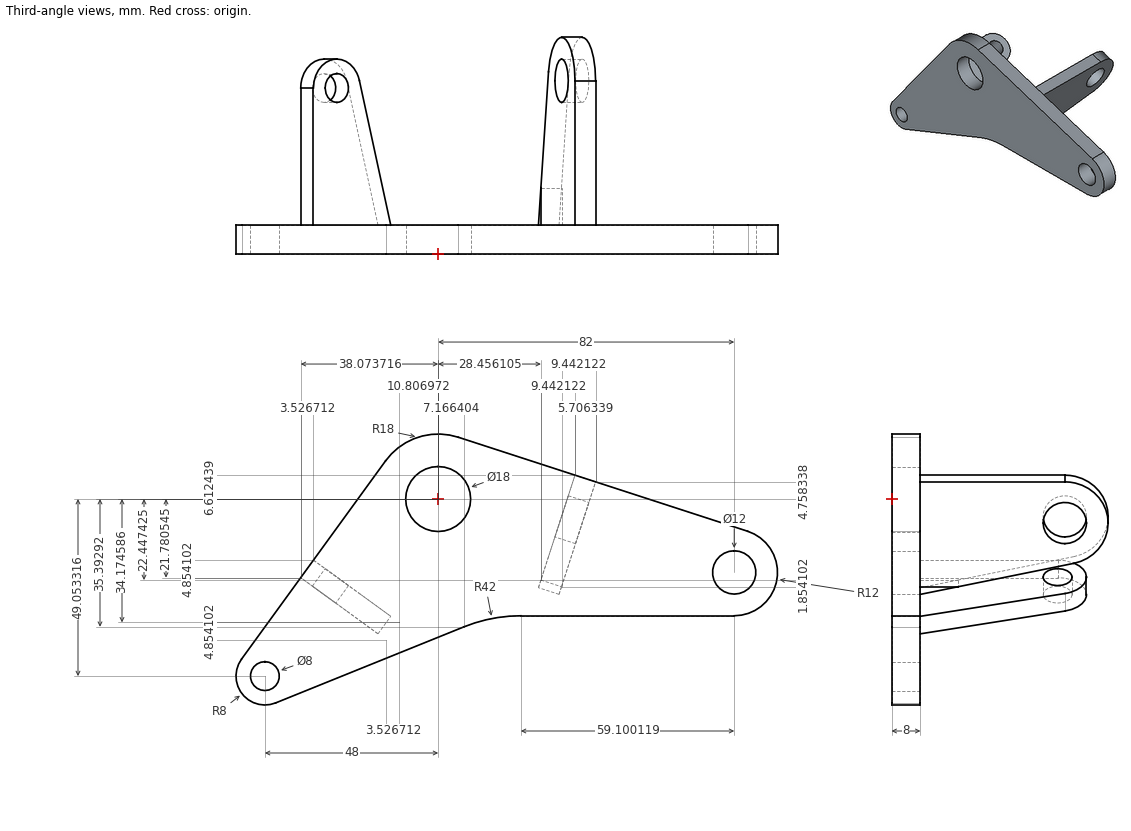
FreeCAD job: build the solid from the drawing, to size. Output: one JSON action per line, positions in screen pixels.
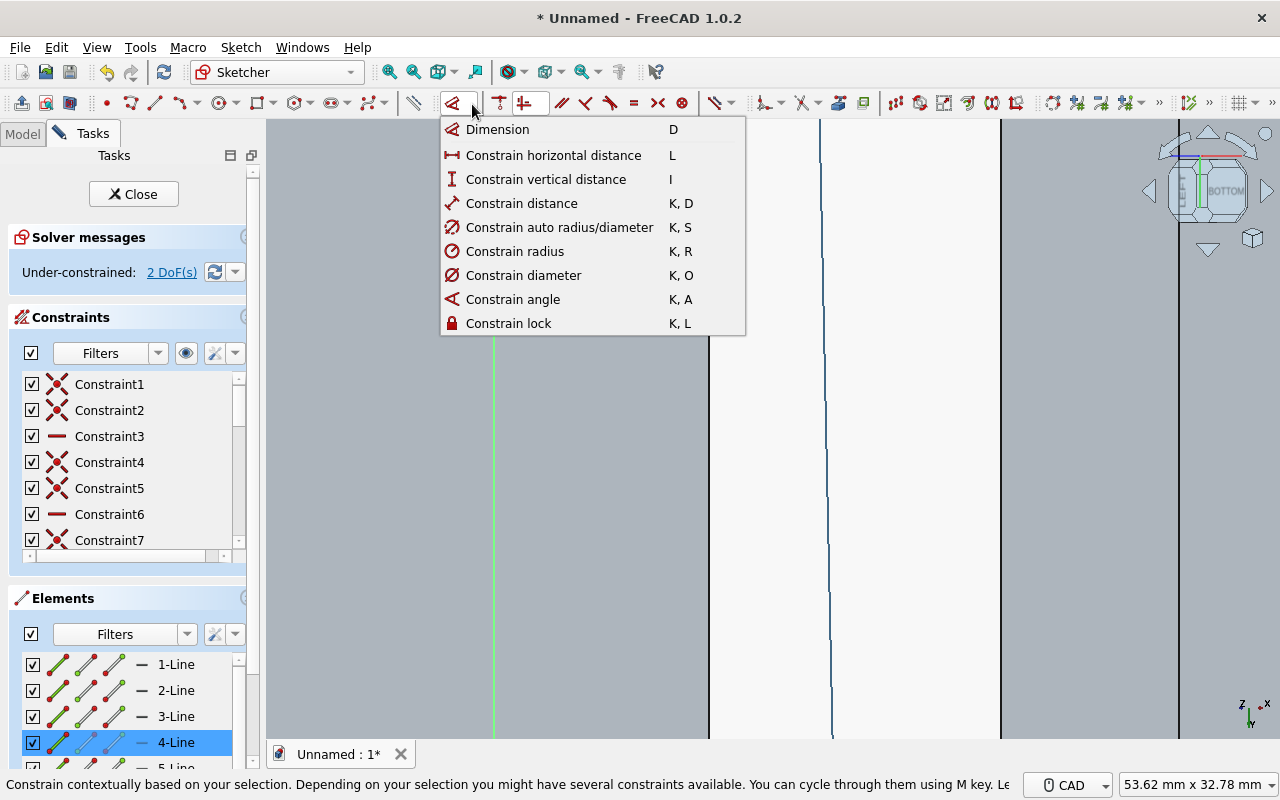
{"action": "left_click", "coordinate": [593, 155]}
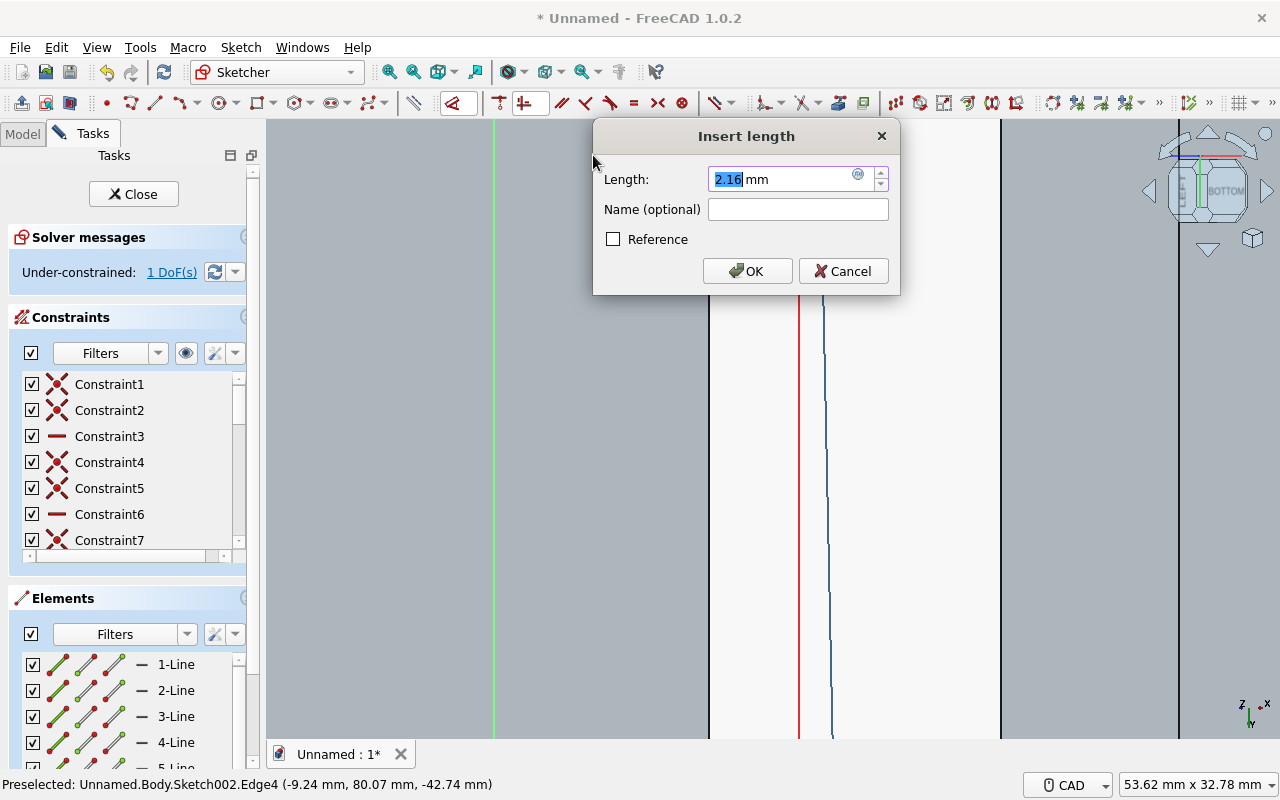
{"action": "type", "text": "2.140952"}
{"action": "key", "text": "Return"}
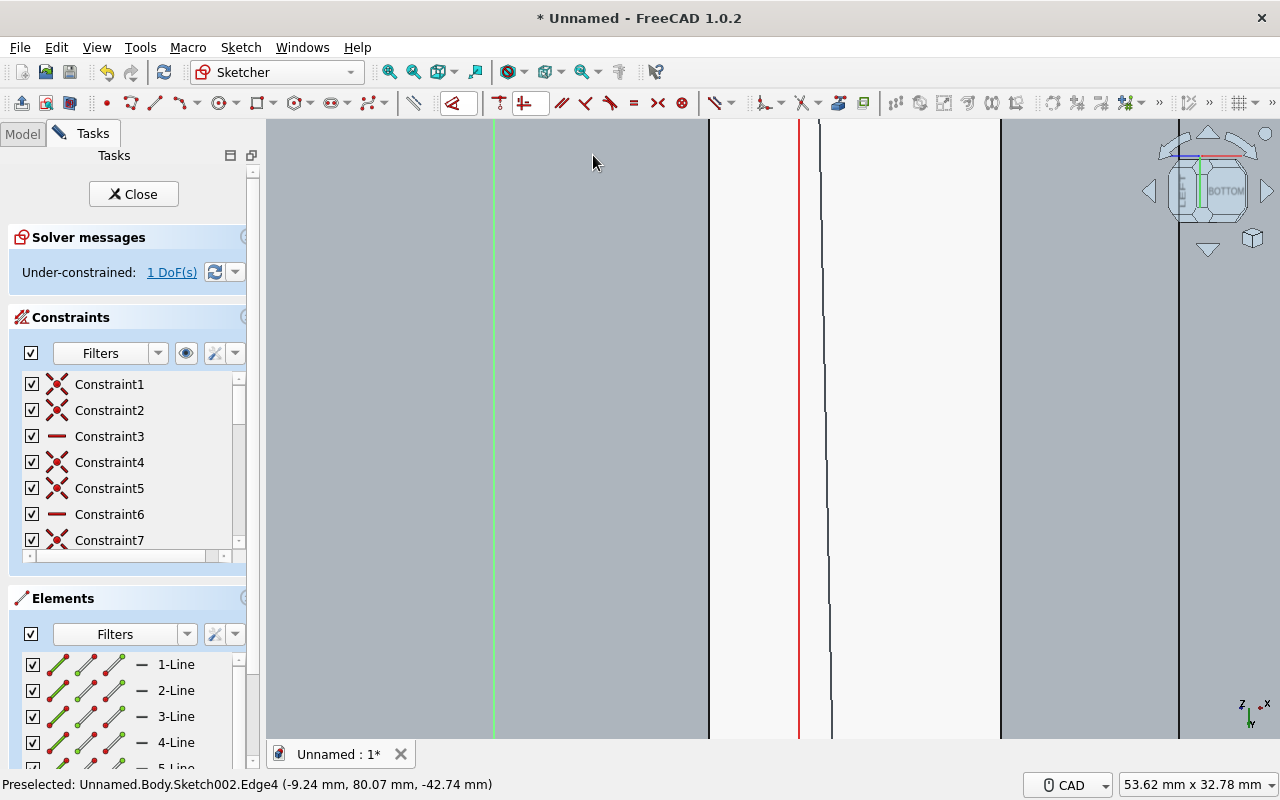
{"action": "scroll", "coordinate": [830, 525], "scroll_direction": "down", "scroll_amount": 8}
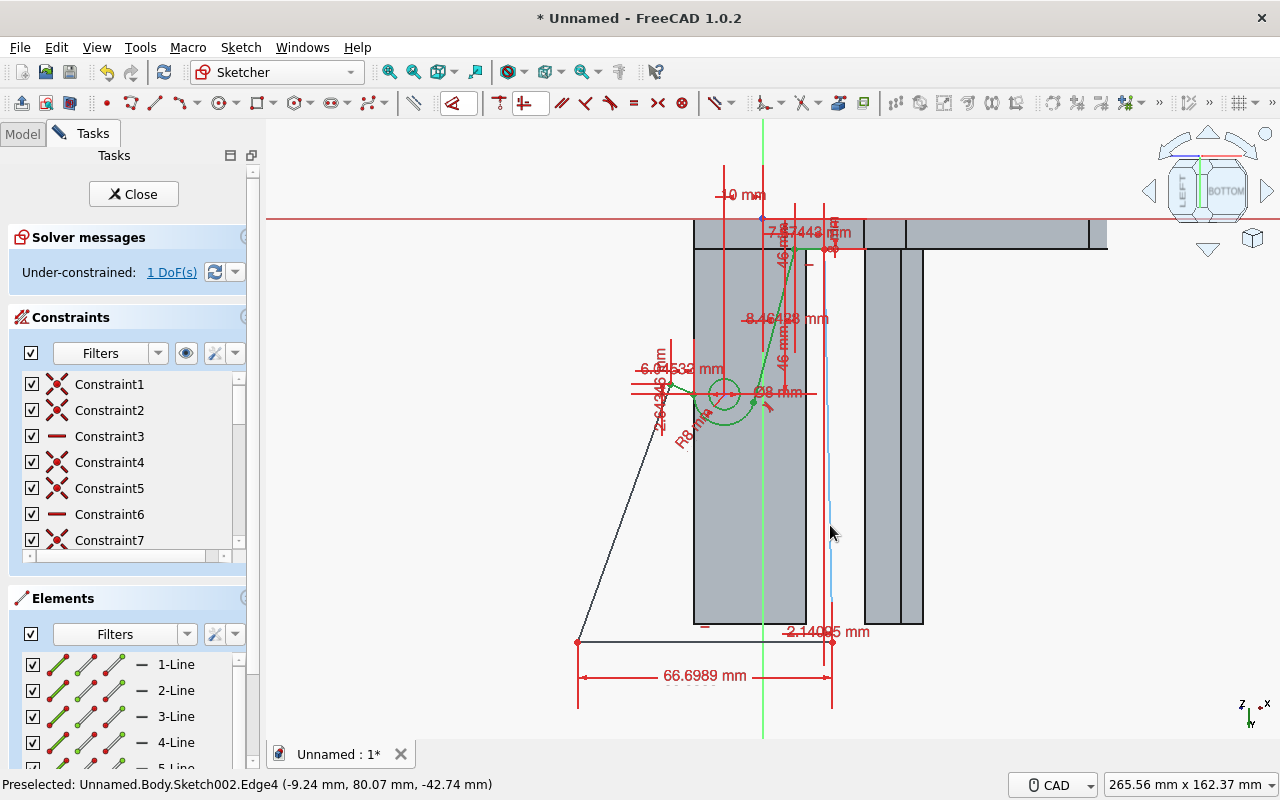
{"action": "left_click", "coordinate": [643, 462]}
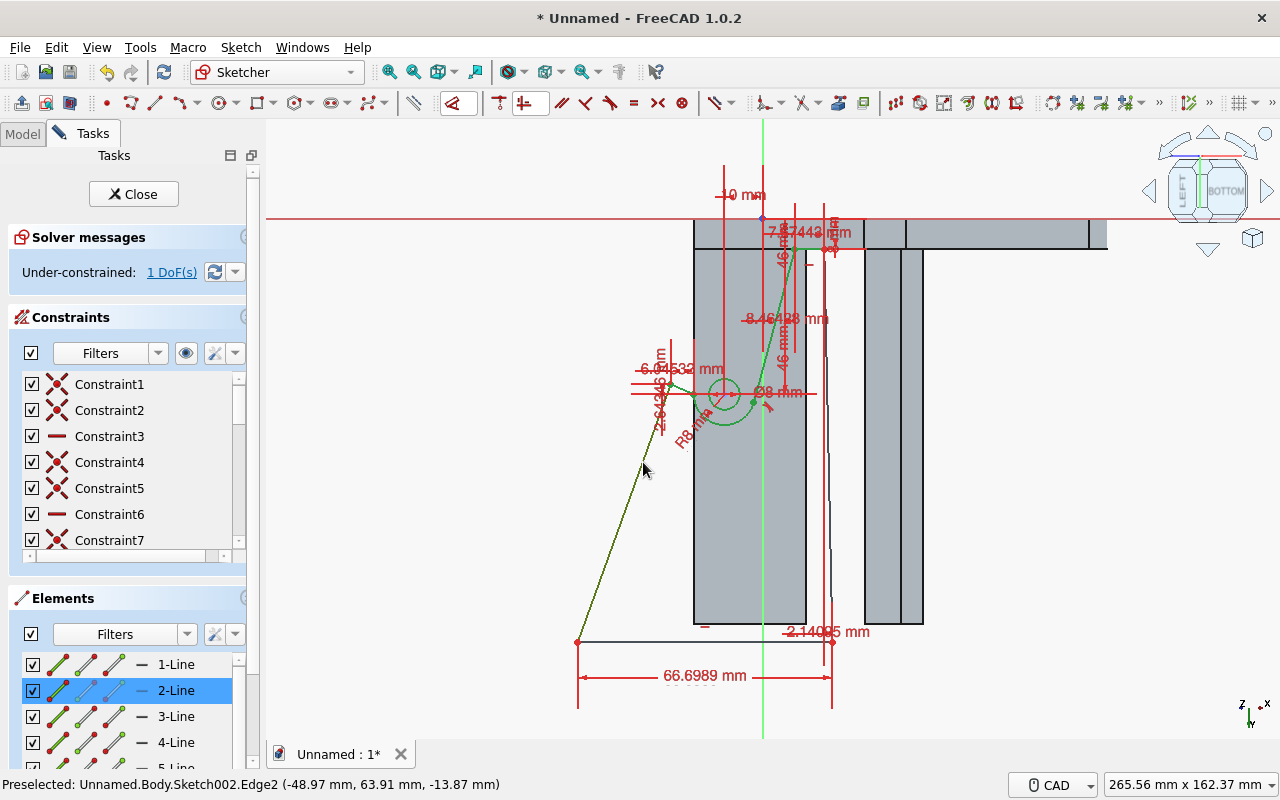
{"action": "left_click", "coordinate": [472, 104]}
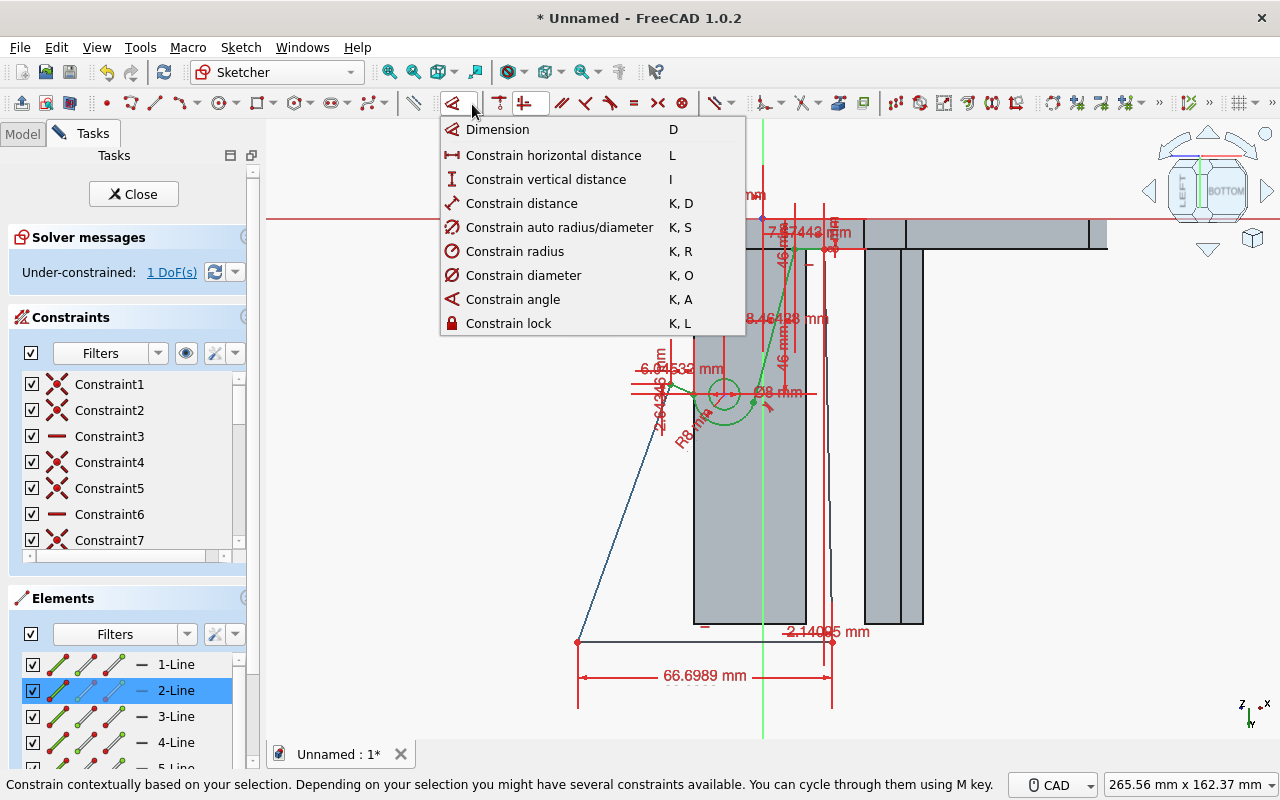
{"action": "left_click", "coordinate": [593, 179]}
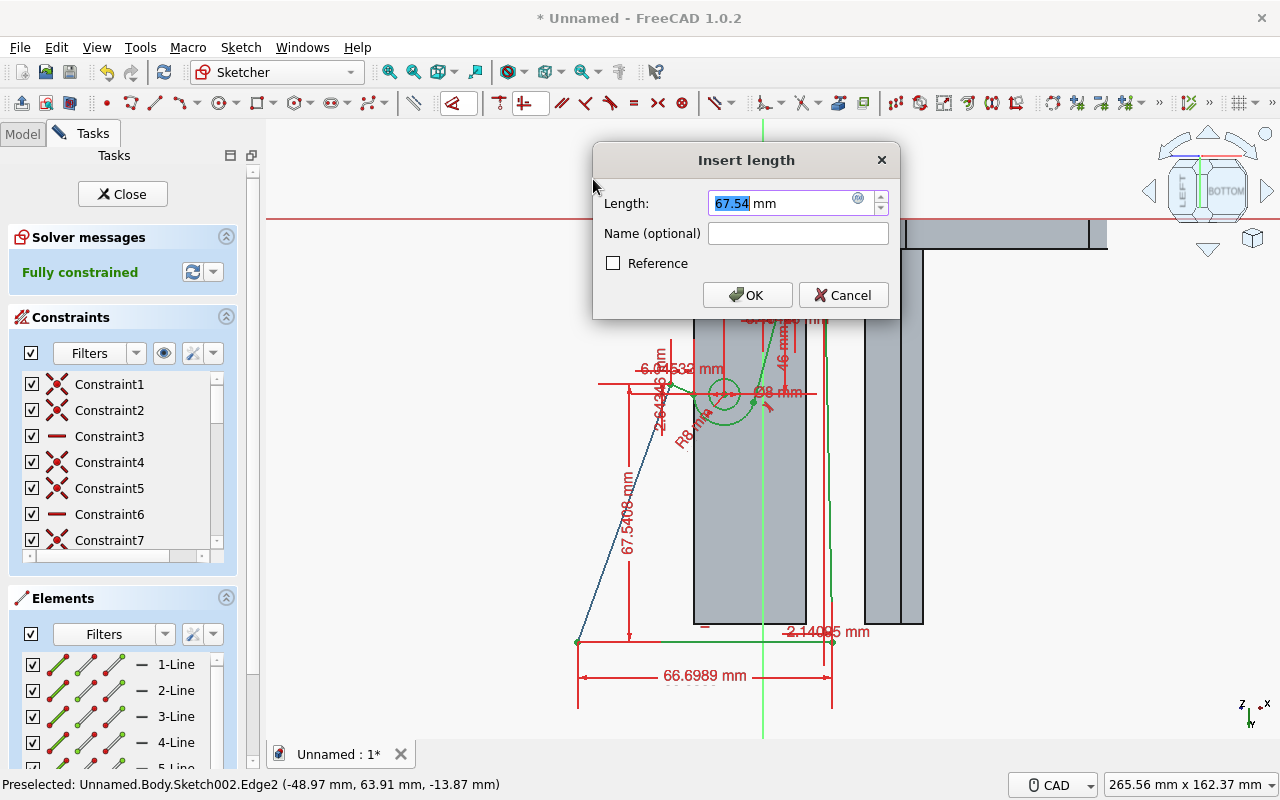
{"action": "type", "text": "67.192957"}
{"action": "key", "text": "Return"}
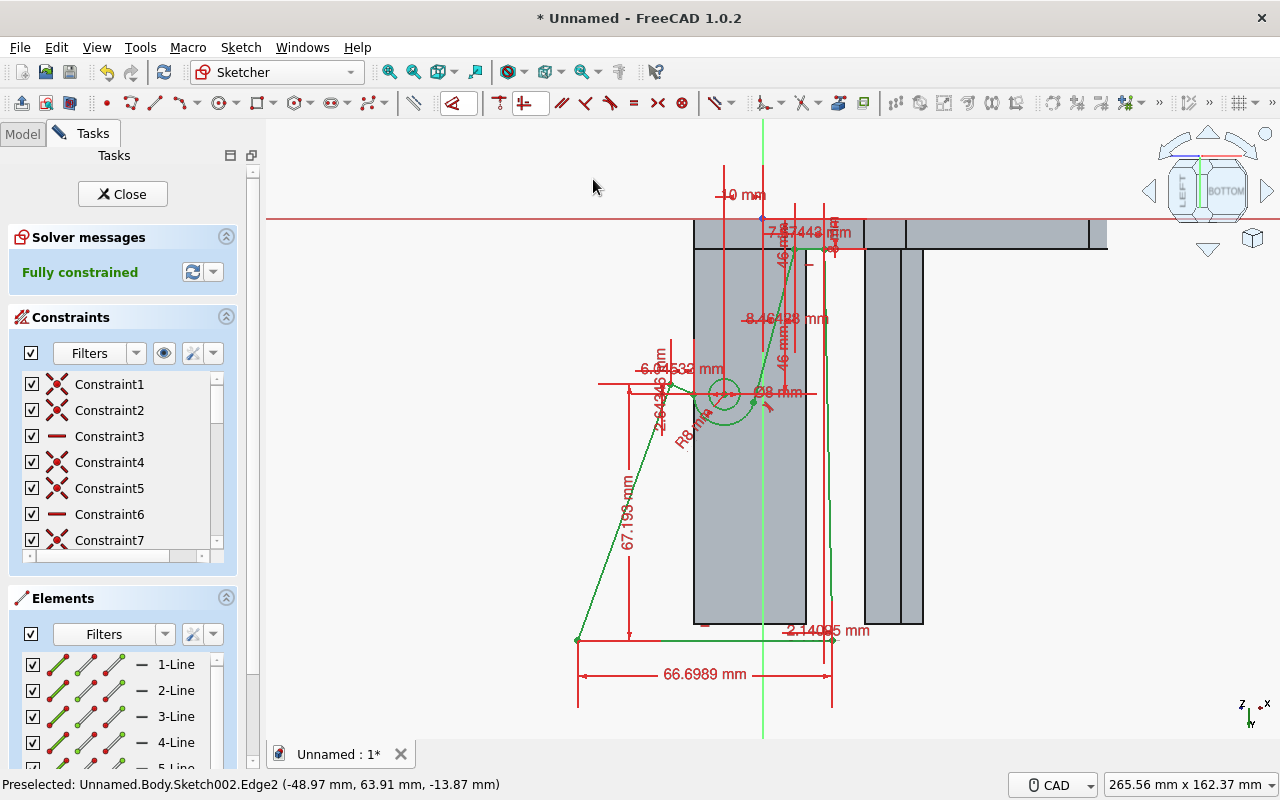
{"action": "left_click", "coordinate": [123, 194]}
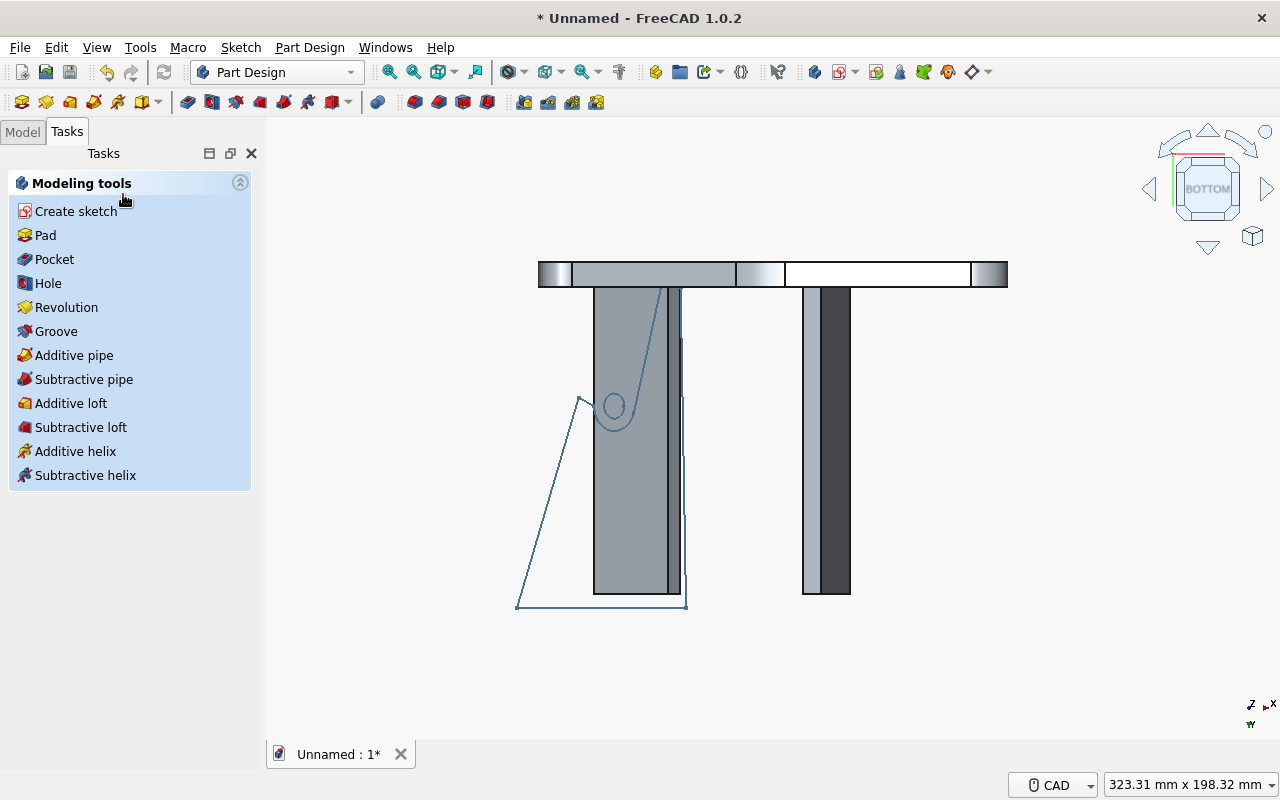
{"action": "left_click", "coordinate": [188, 102]}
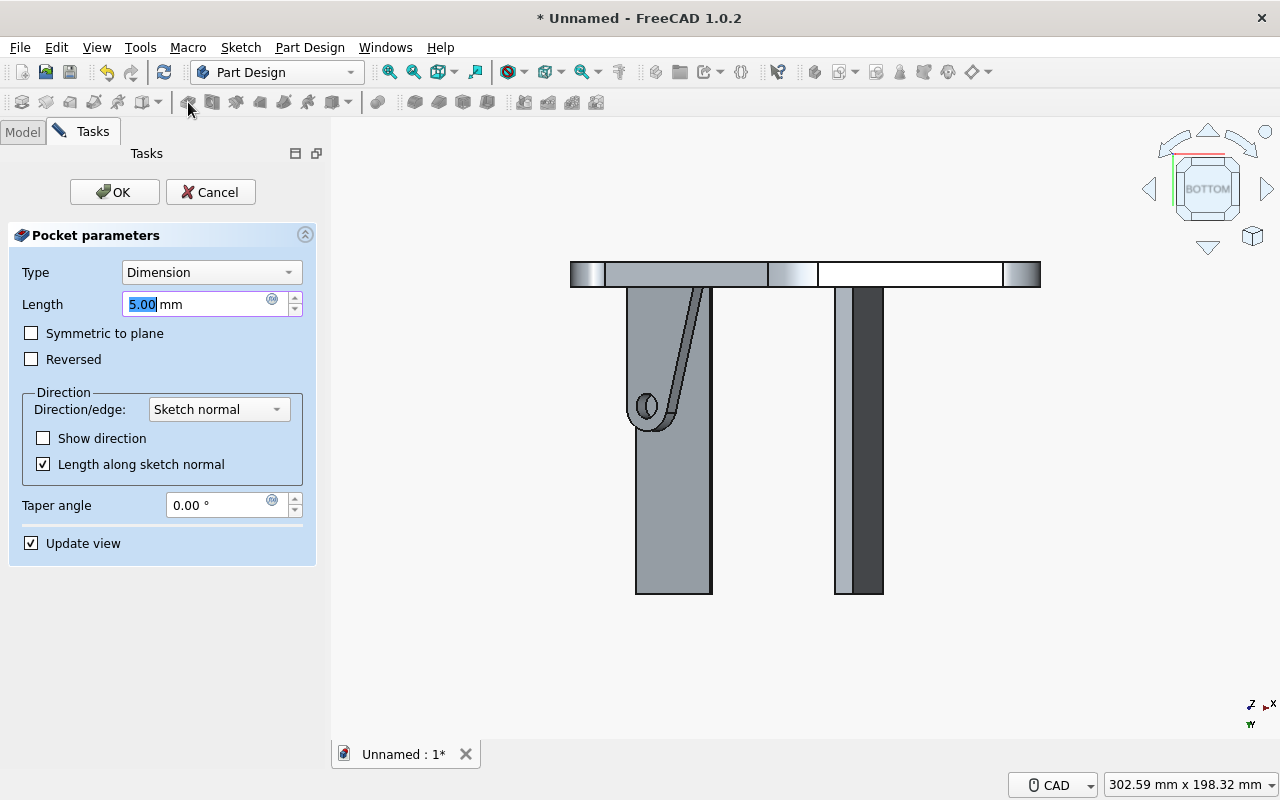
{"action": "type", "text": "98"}
{"action": "key", "text": "Tab"}